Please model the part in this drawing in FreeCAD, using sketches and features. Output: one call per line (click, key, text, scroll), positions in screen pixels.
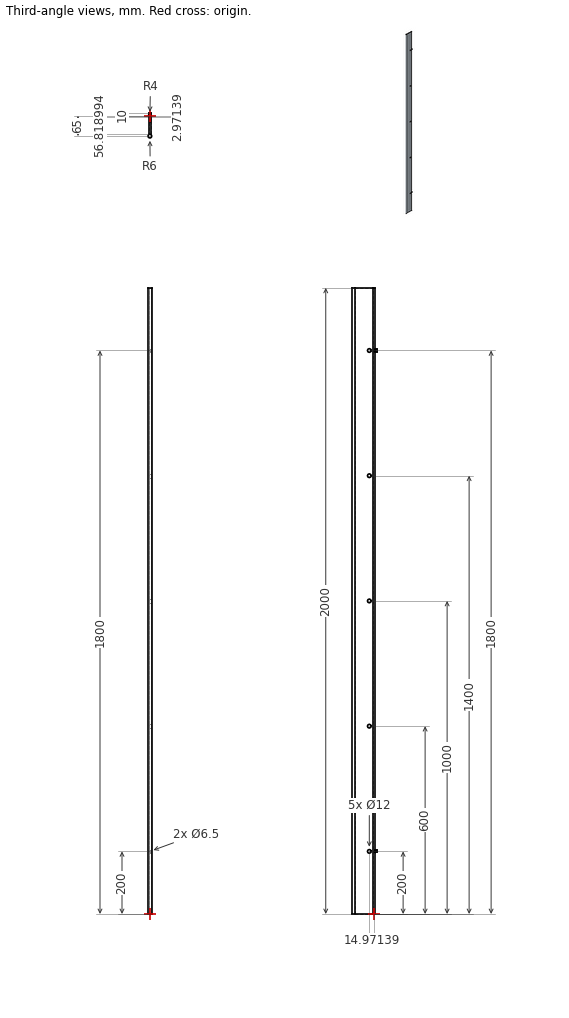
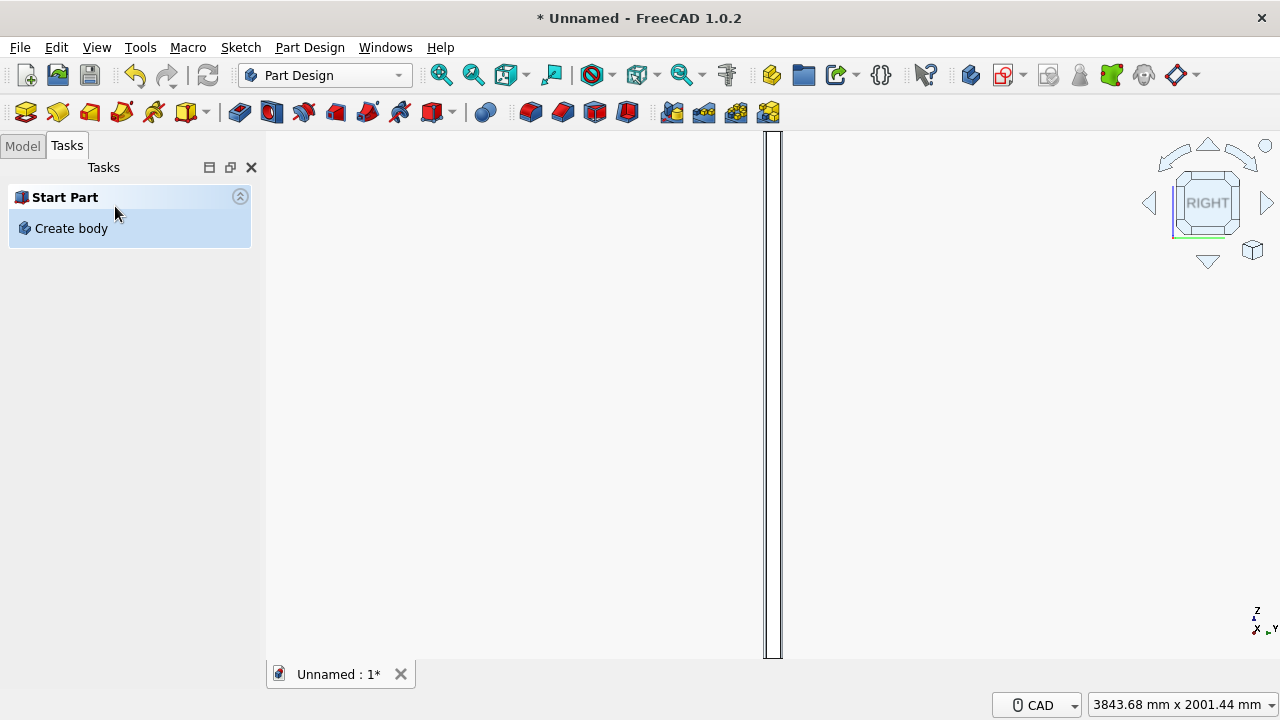
key(2)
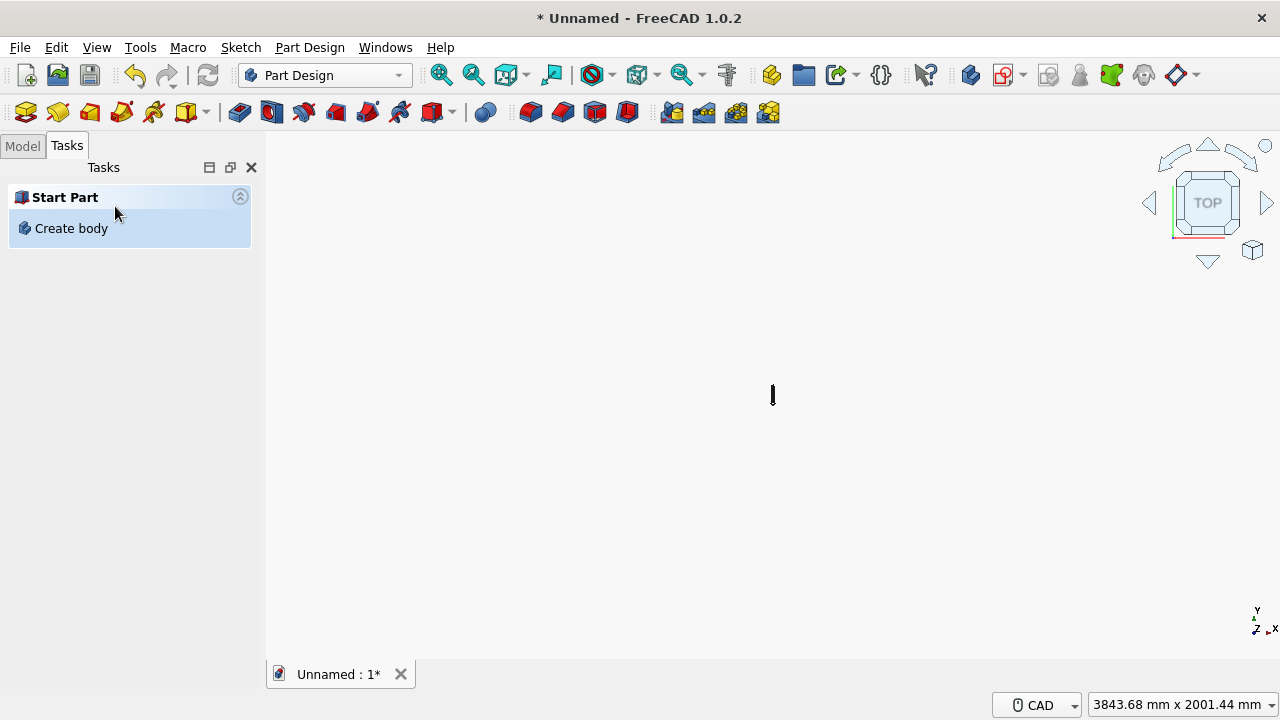
key(v)
key(f)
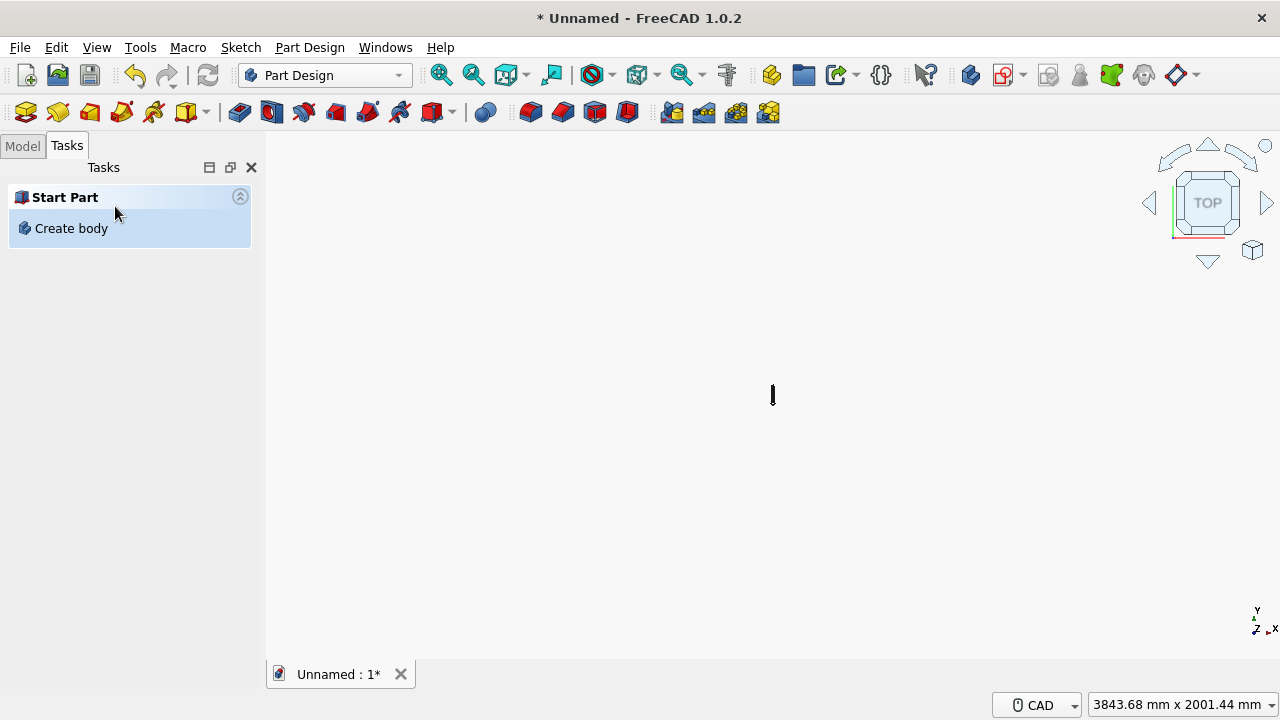
click(23, 145)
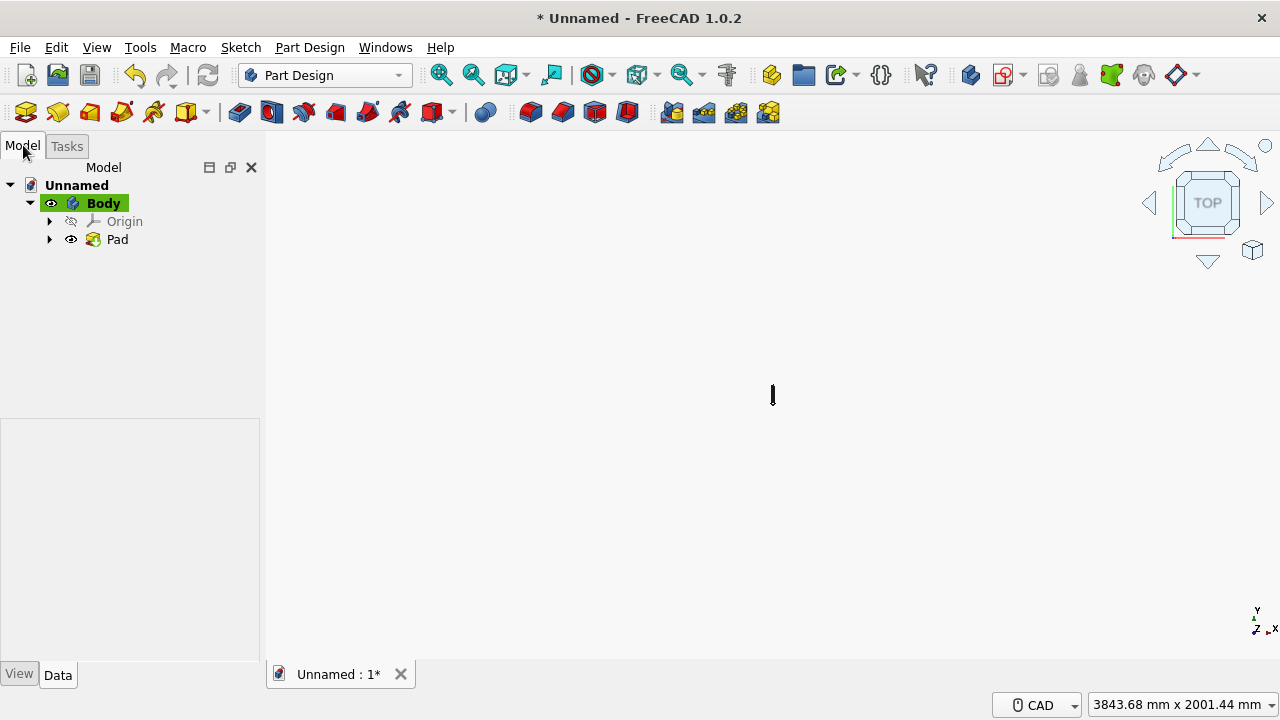
click(50, 221)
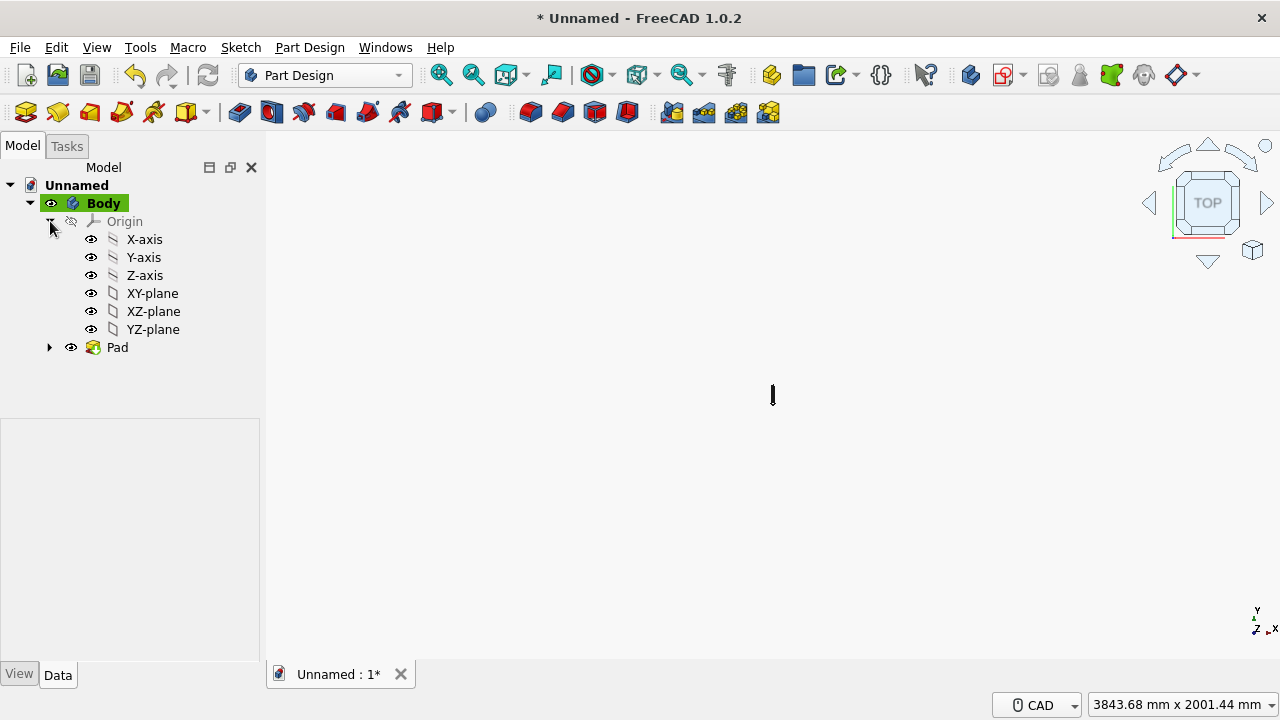
click(136, 329)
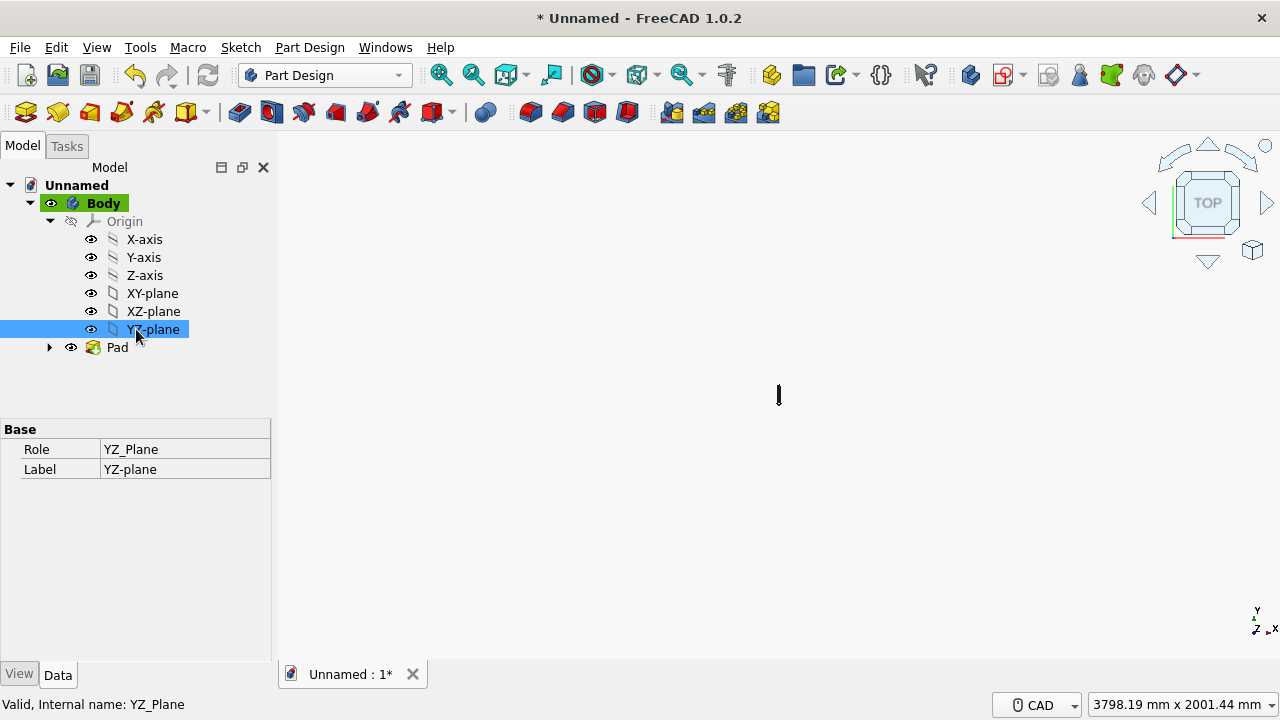
click(1176, 76)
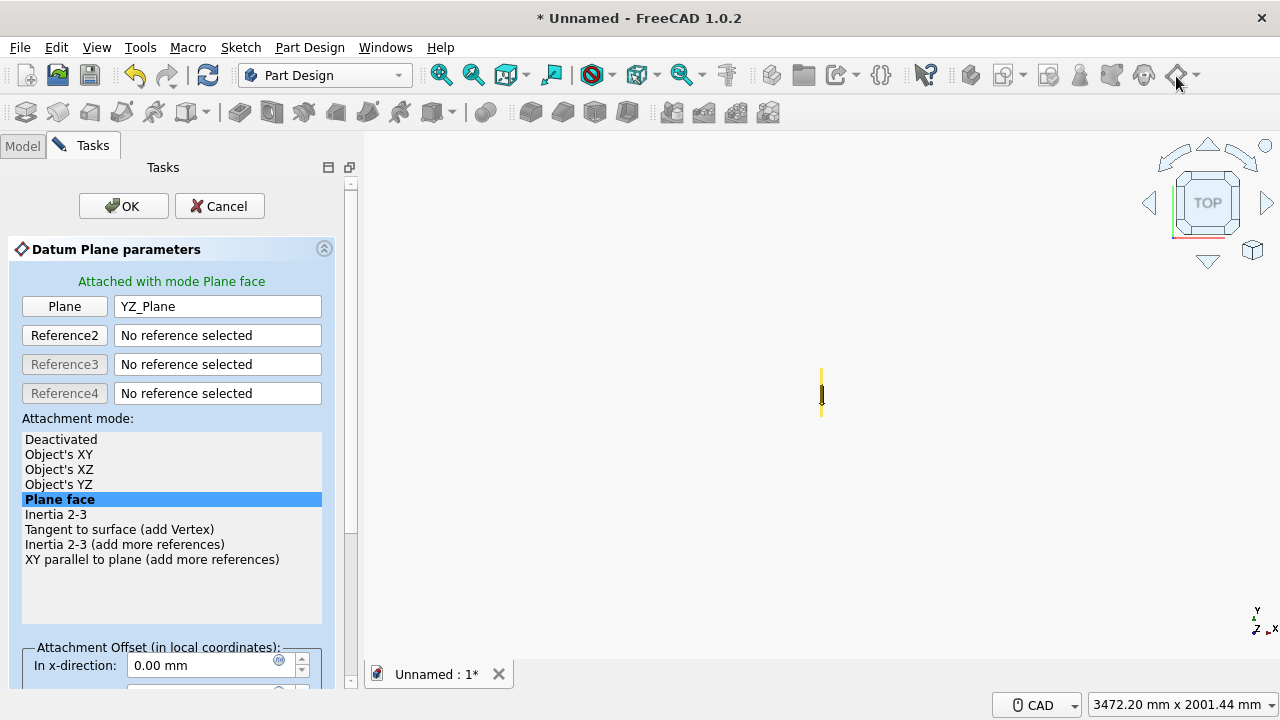
scroll(351, 432, down, 2)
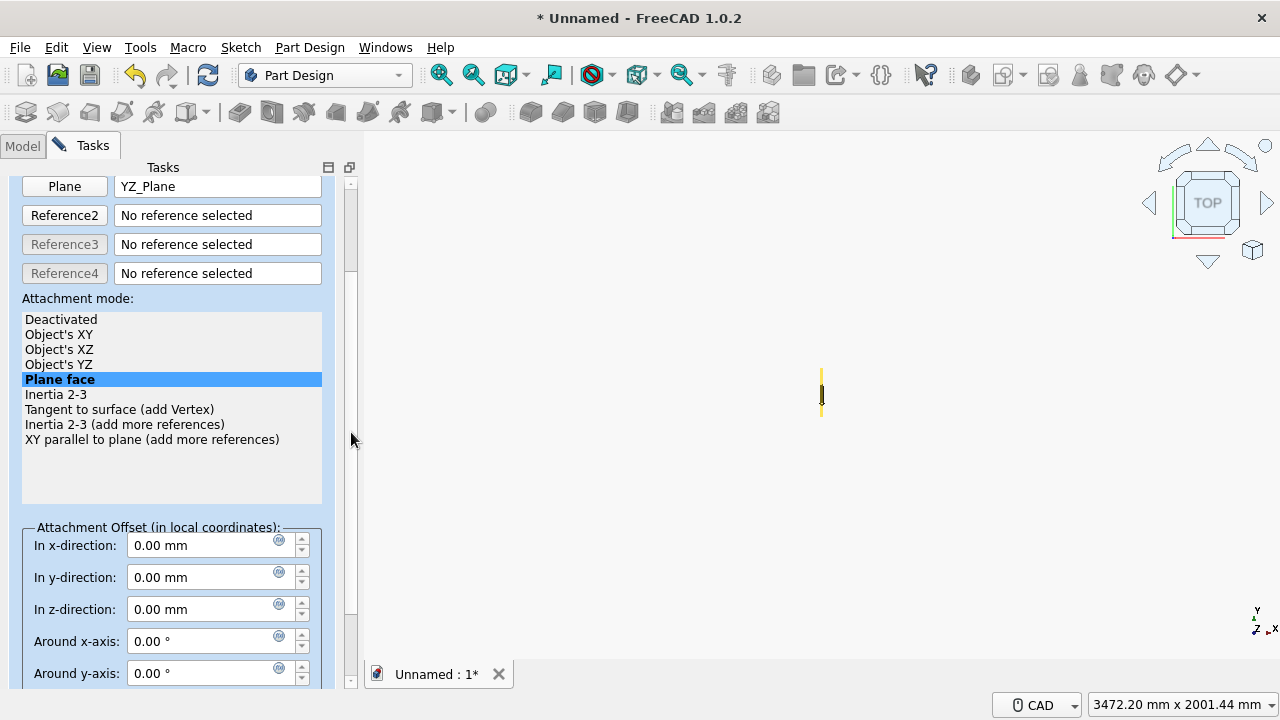
triple_click(210, 609)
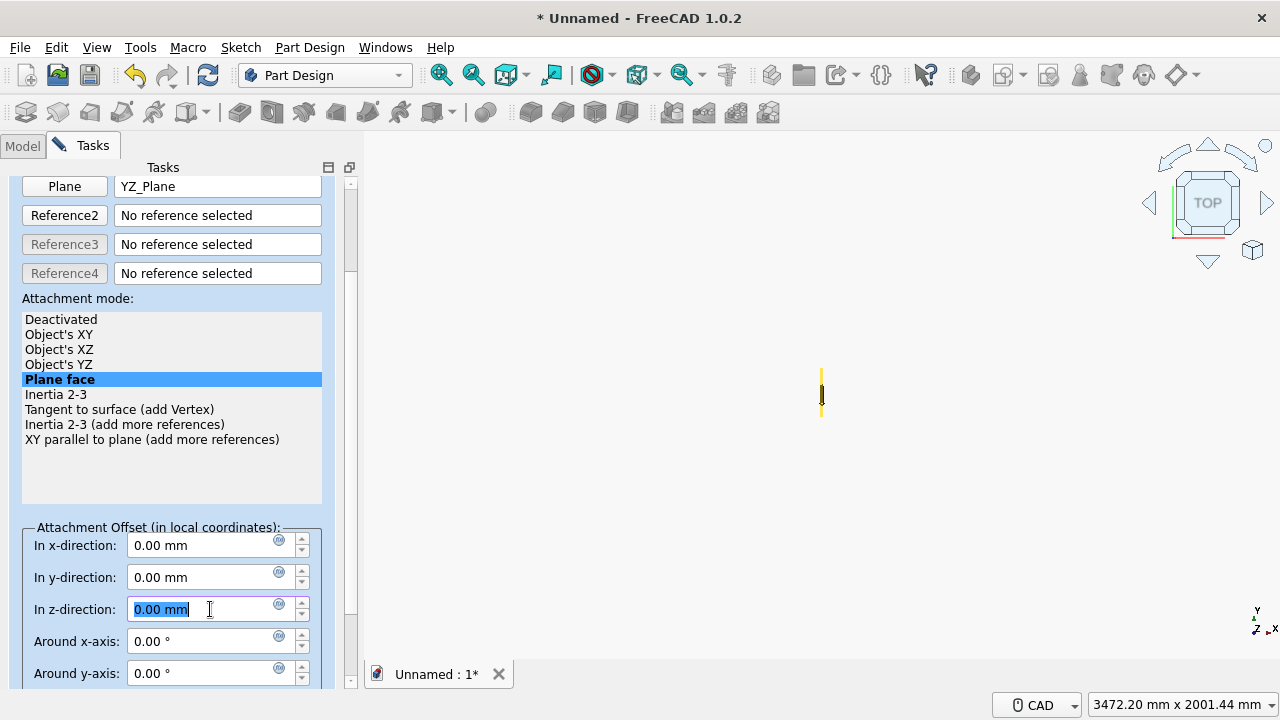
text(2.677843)
key(Tab)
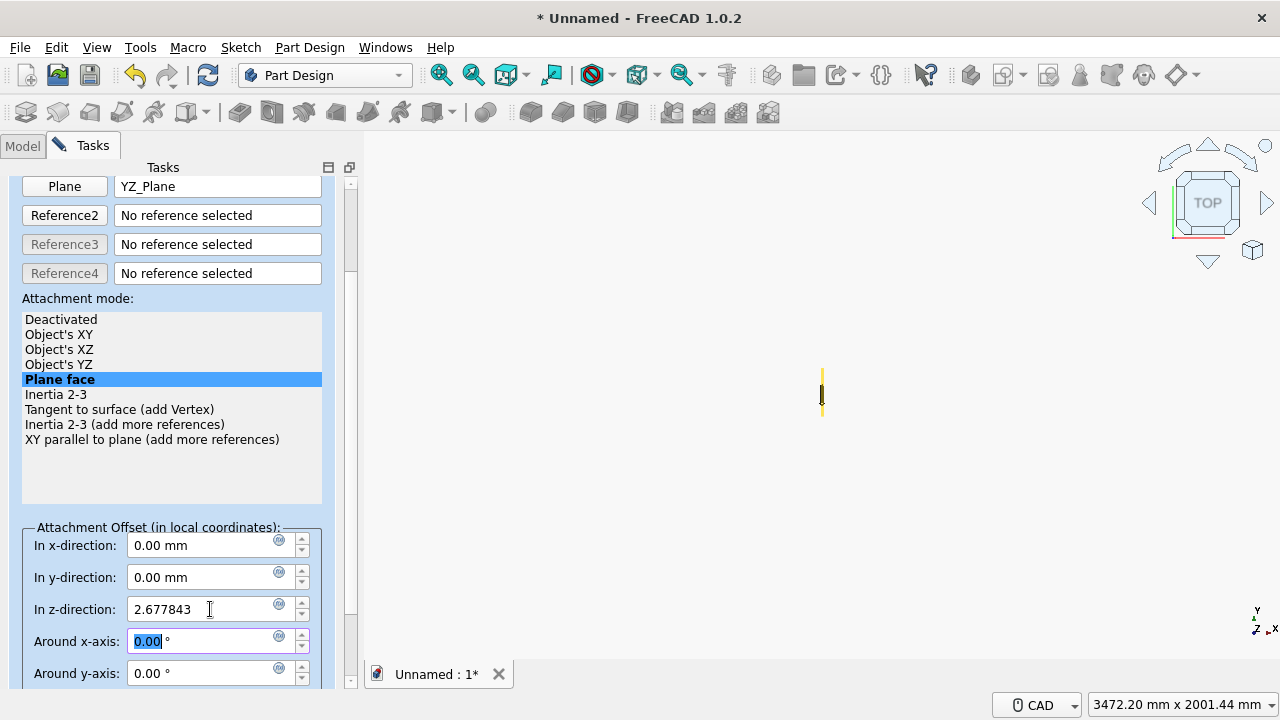
scroll(351, 432, up, 3)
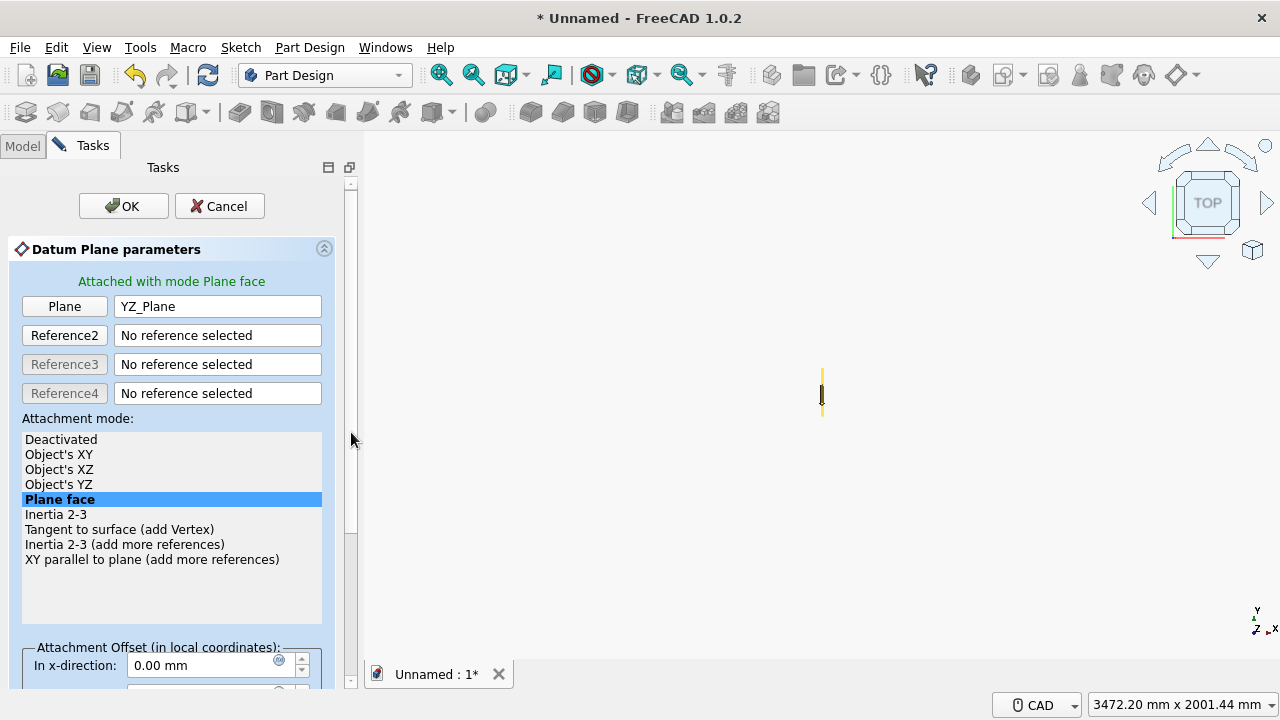
click(124, 206)